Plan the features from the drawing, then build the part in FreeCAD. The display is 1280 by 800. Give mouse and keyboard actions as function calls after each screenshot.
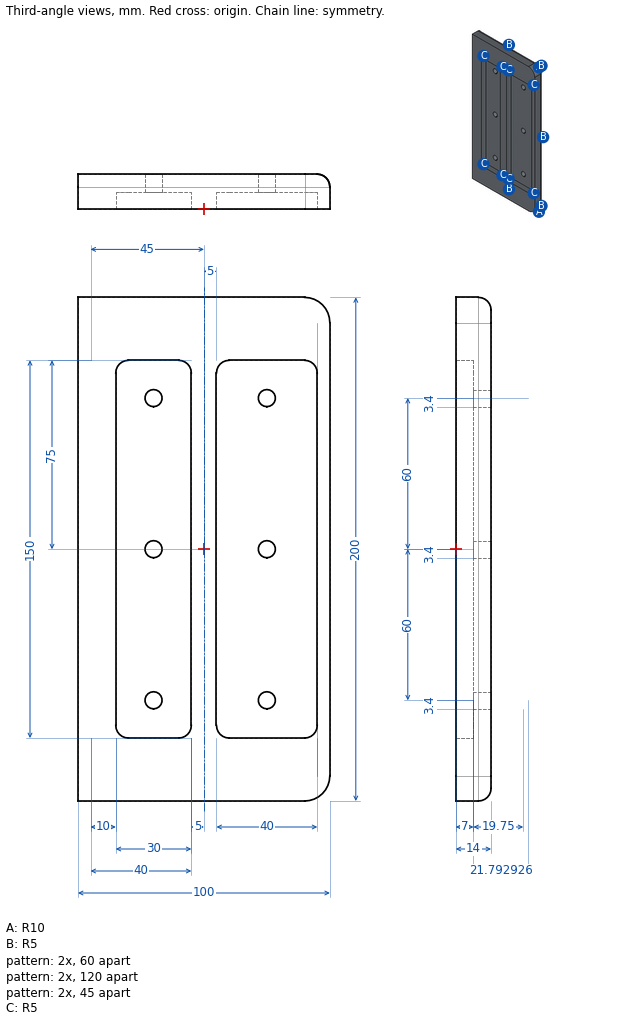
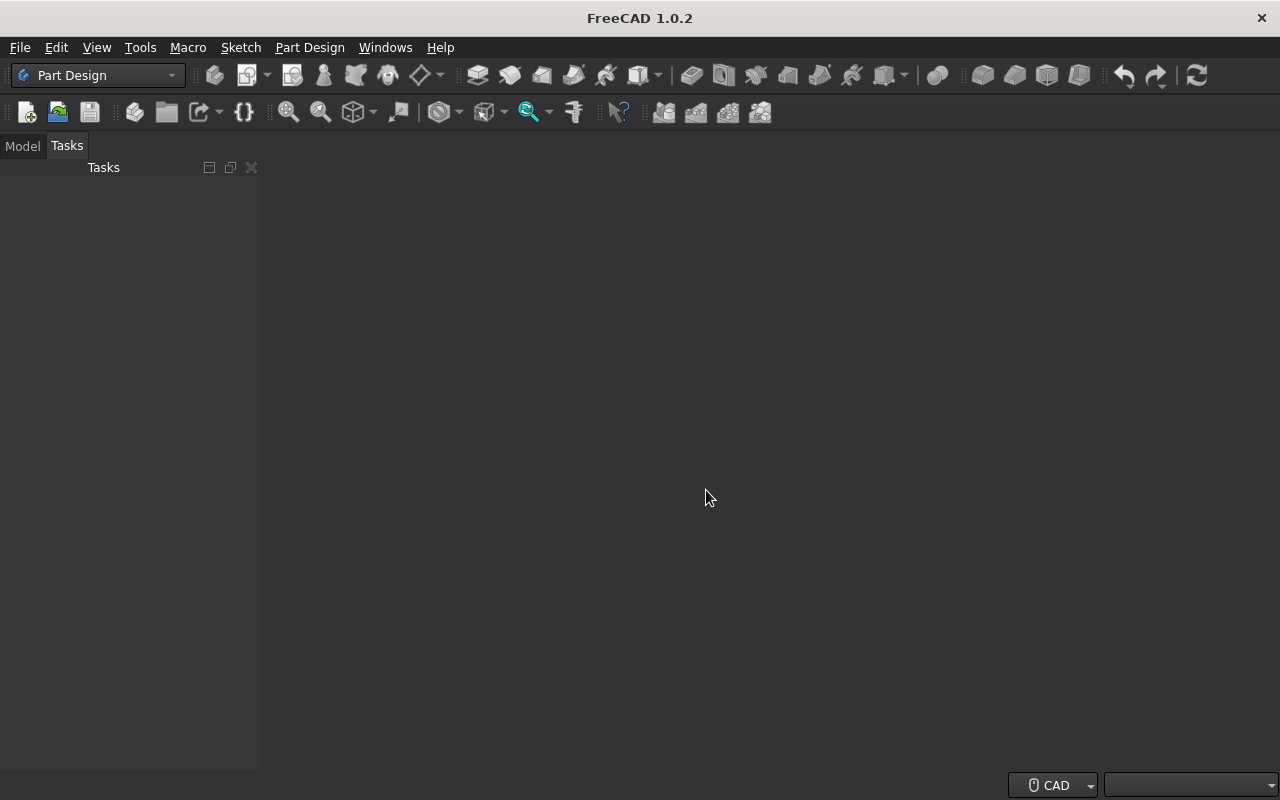
click(26, 112)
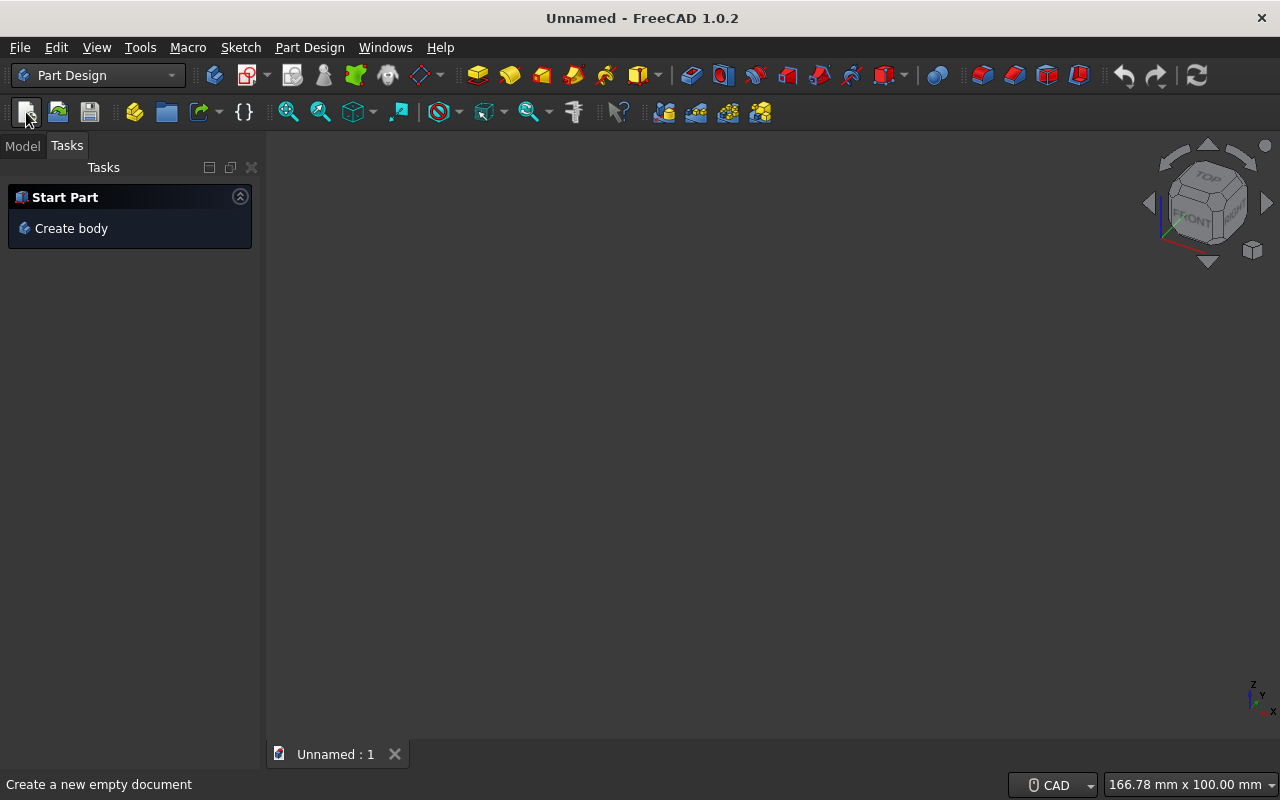
click(248, 76)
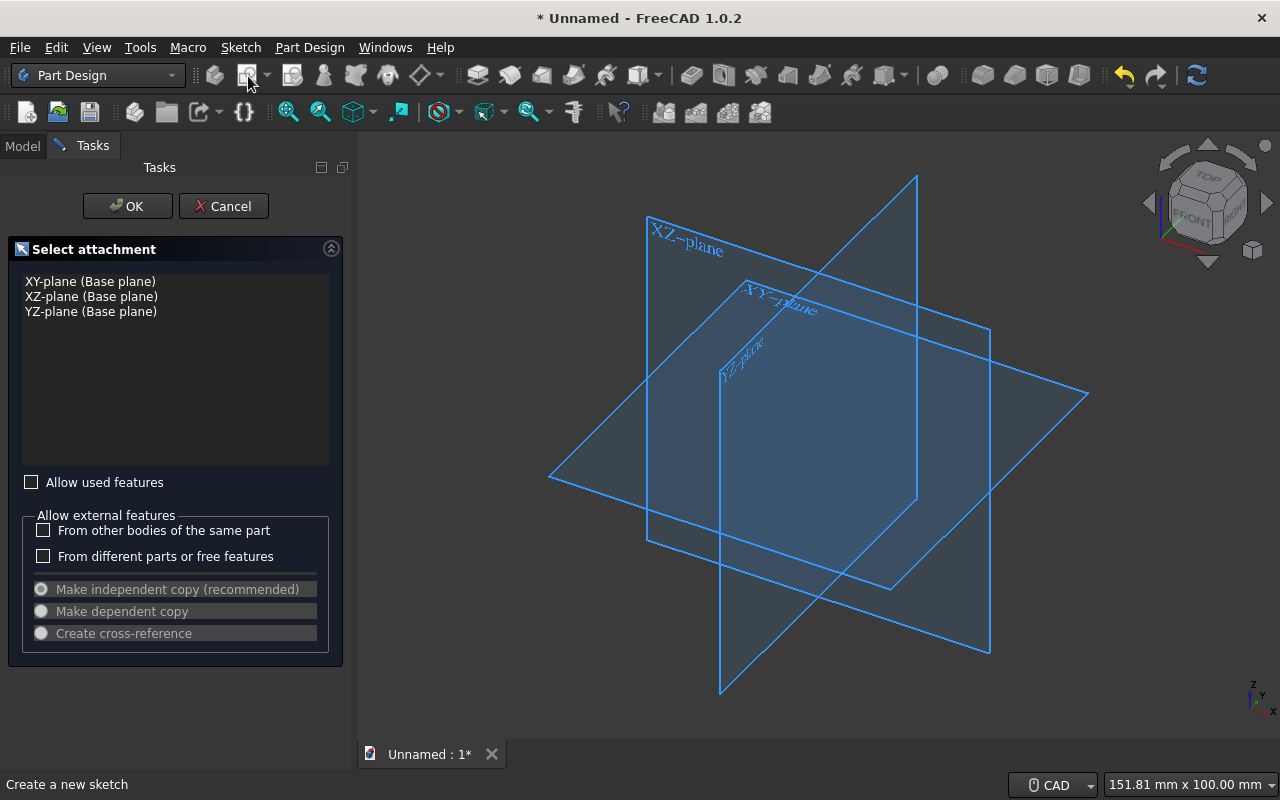
click(82, 296)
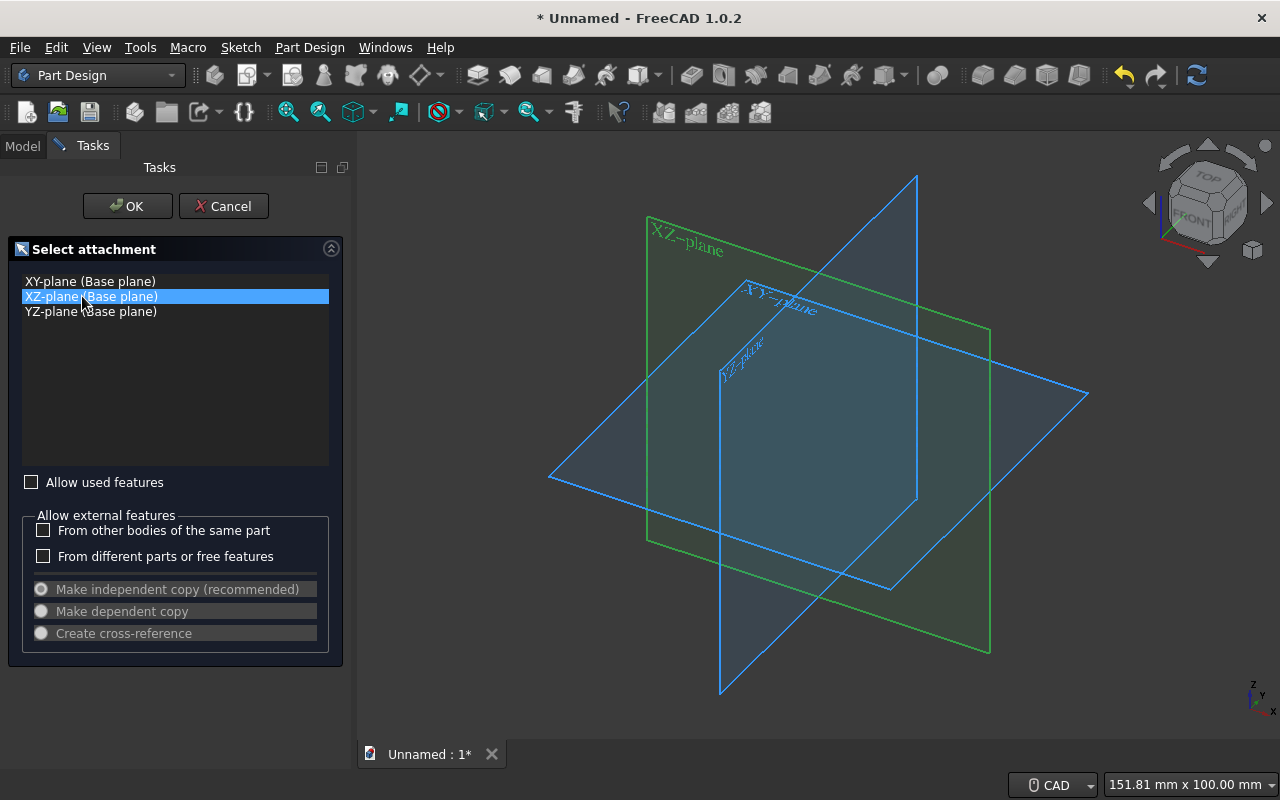
click(128, 206)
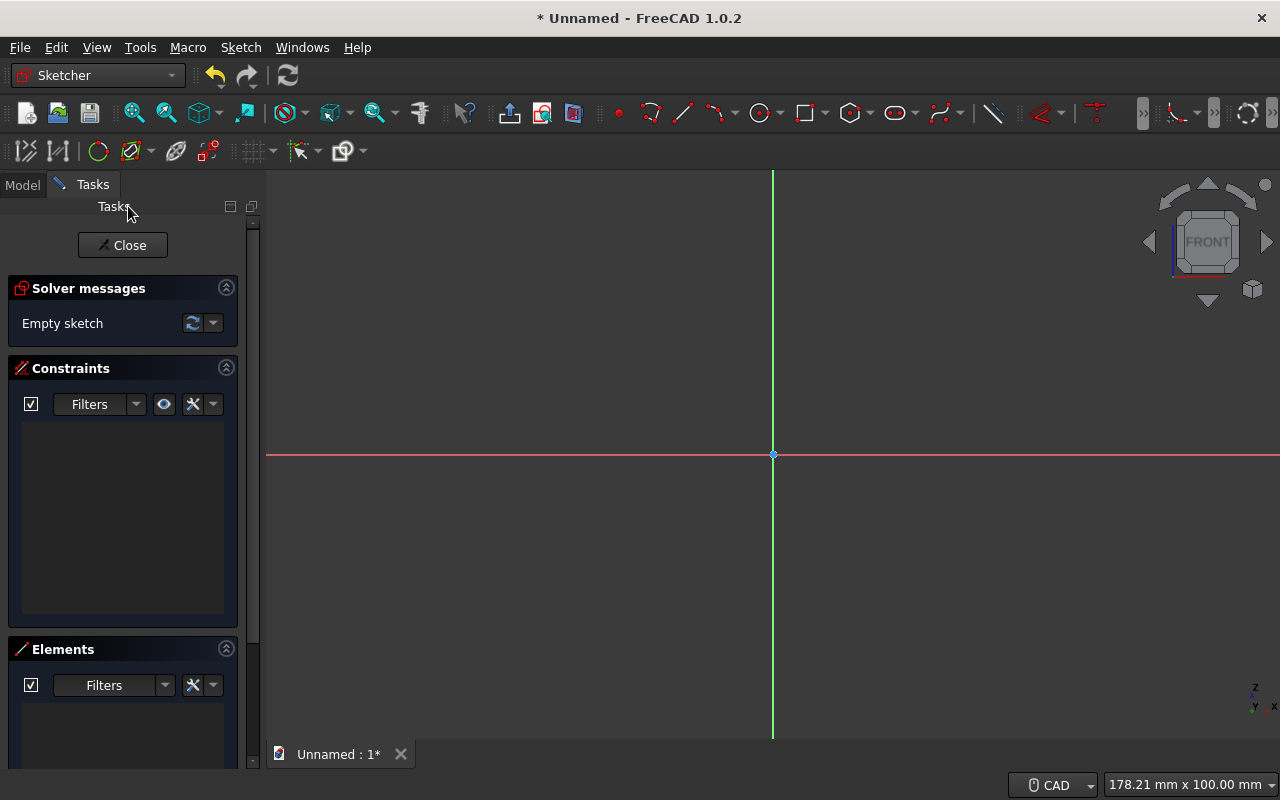
scroll(675, 454, down, 6)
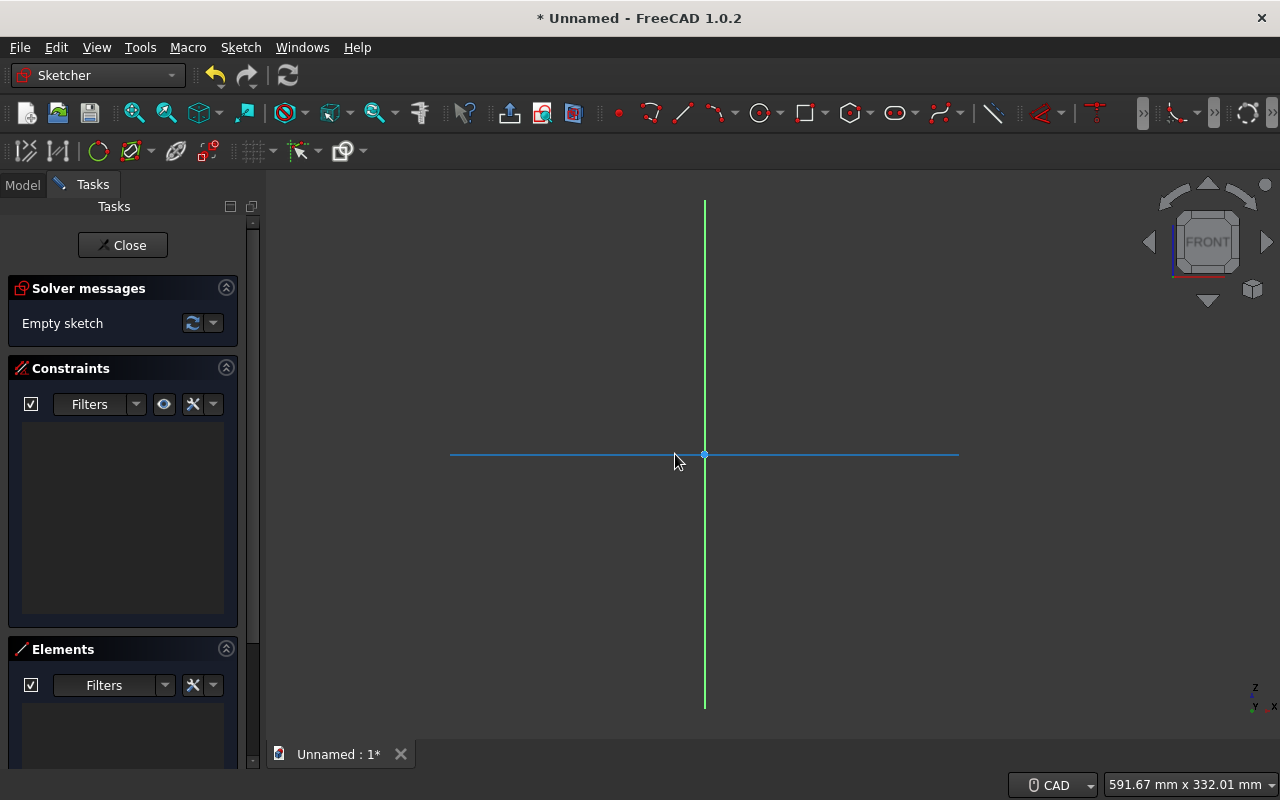
key(g)
key(v)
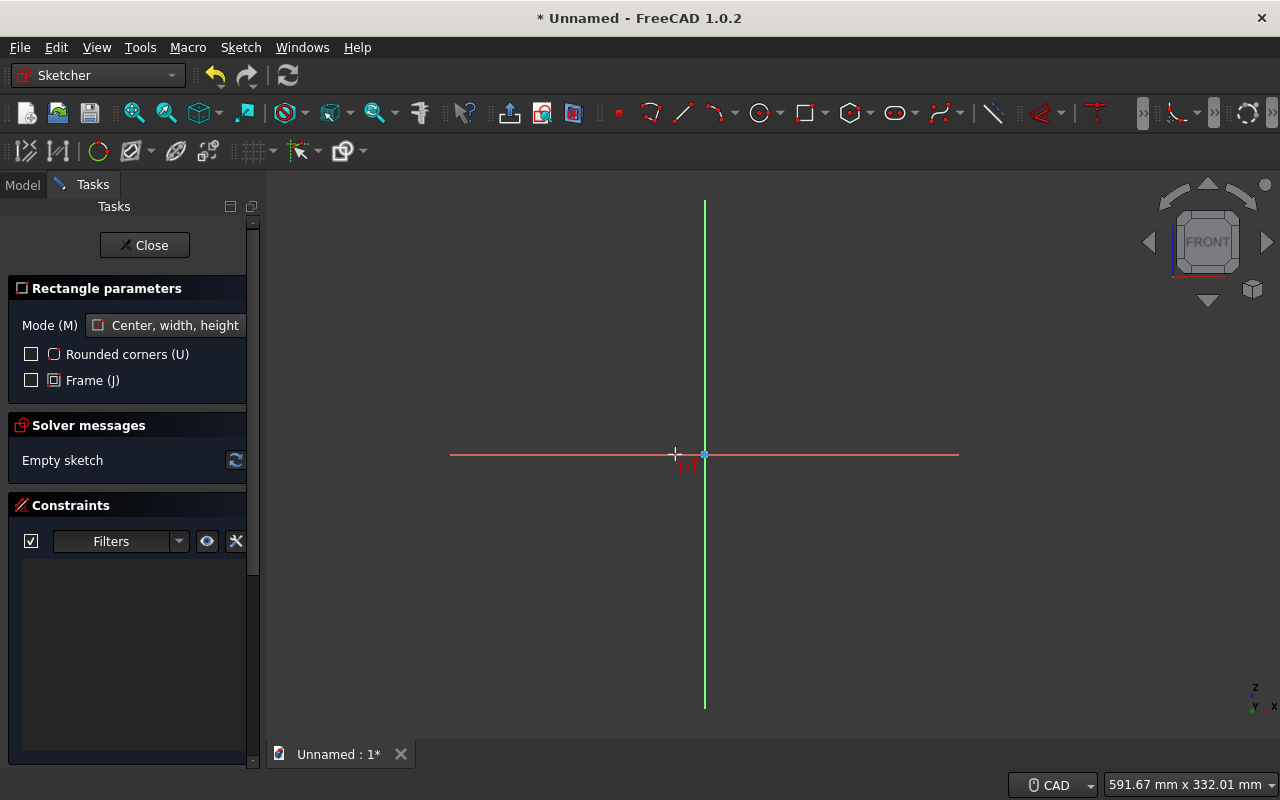
click(705, 454)
move(790, 283)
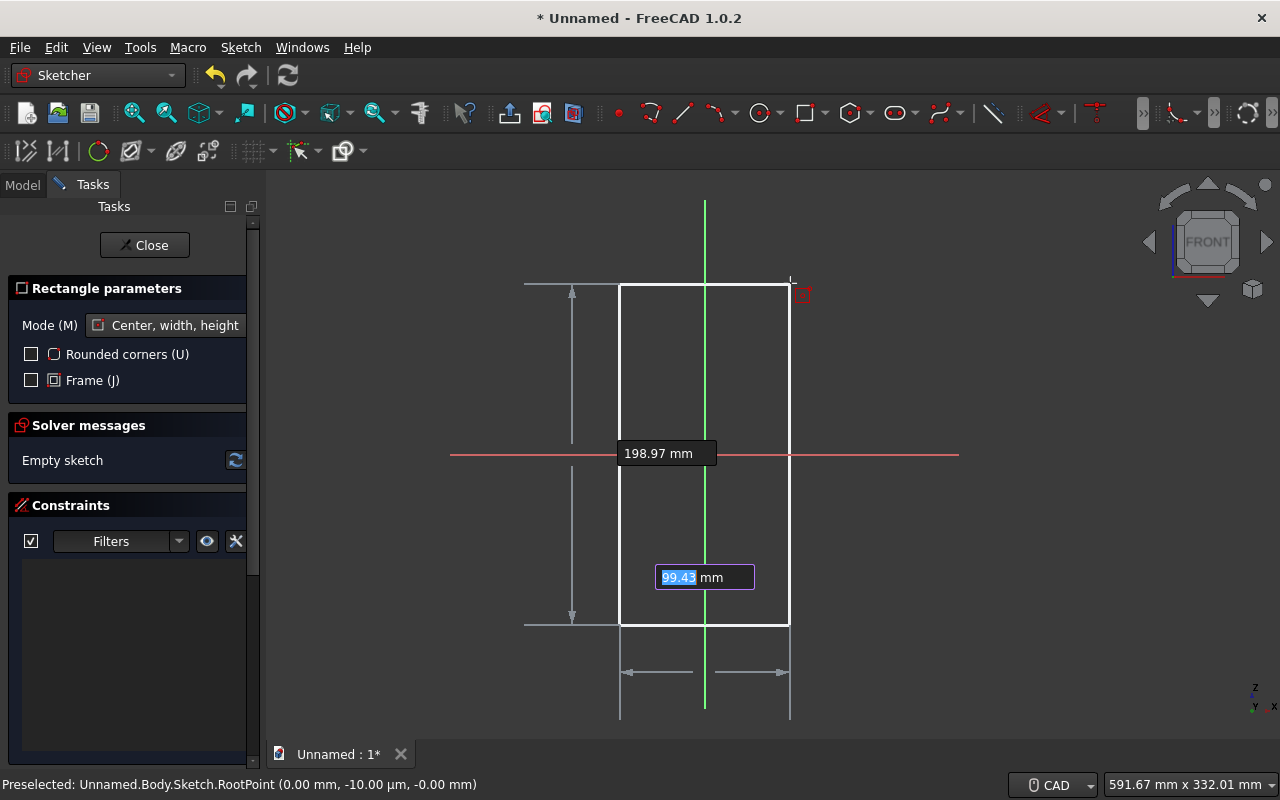
text(100)
key(Tab)
text(200)
key(Return)
key(Escape)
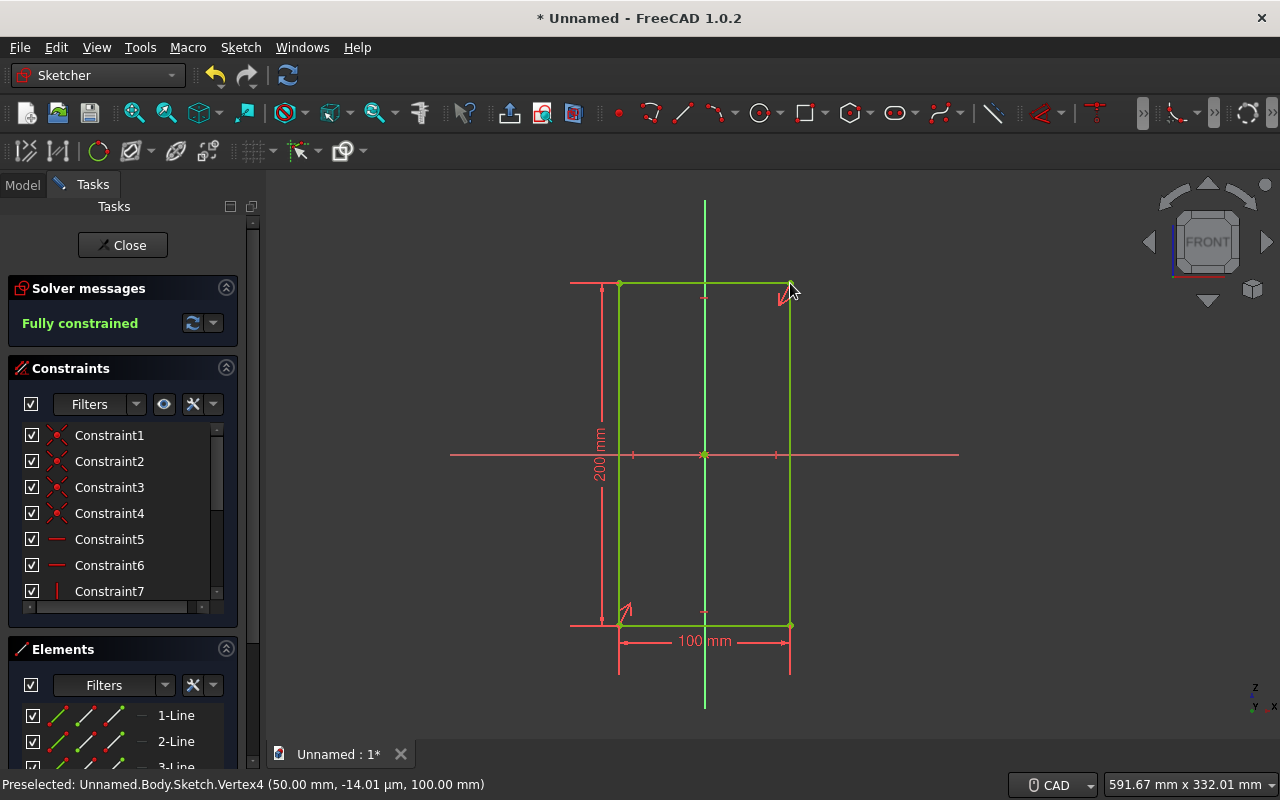
click(123, 245)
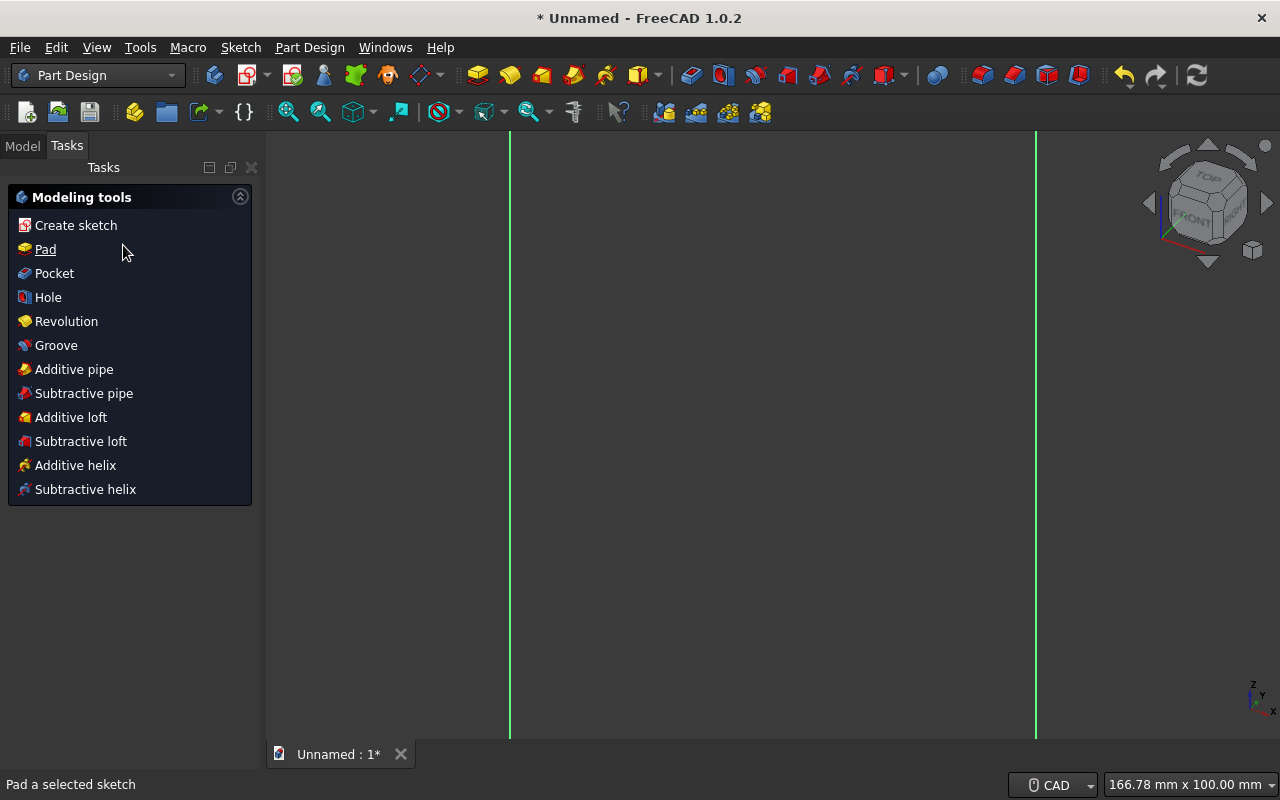
click(478, 76)